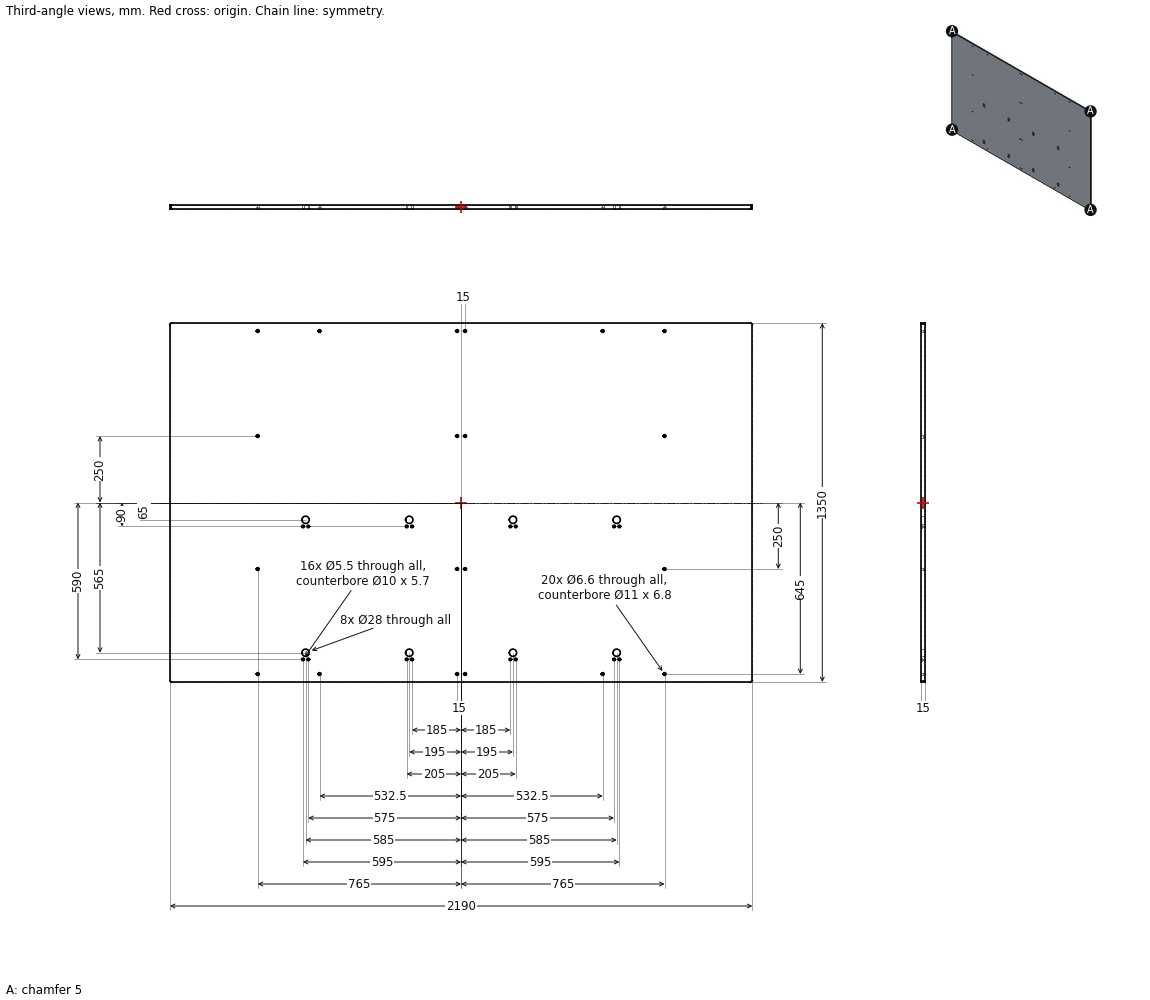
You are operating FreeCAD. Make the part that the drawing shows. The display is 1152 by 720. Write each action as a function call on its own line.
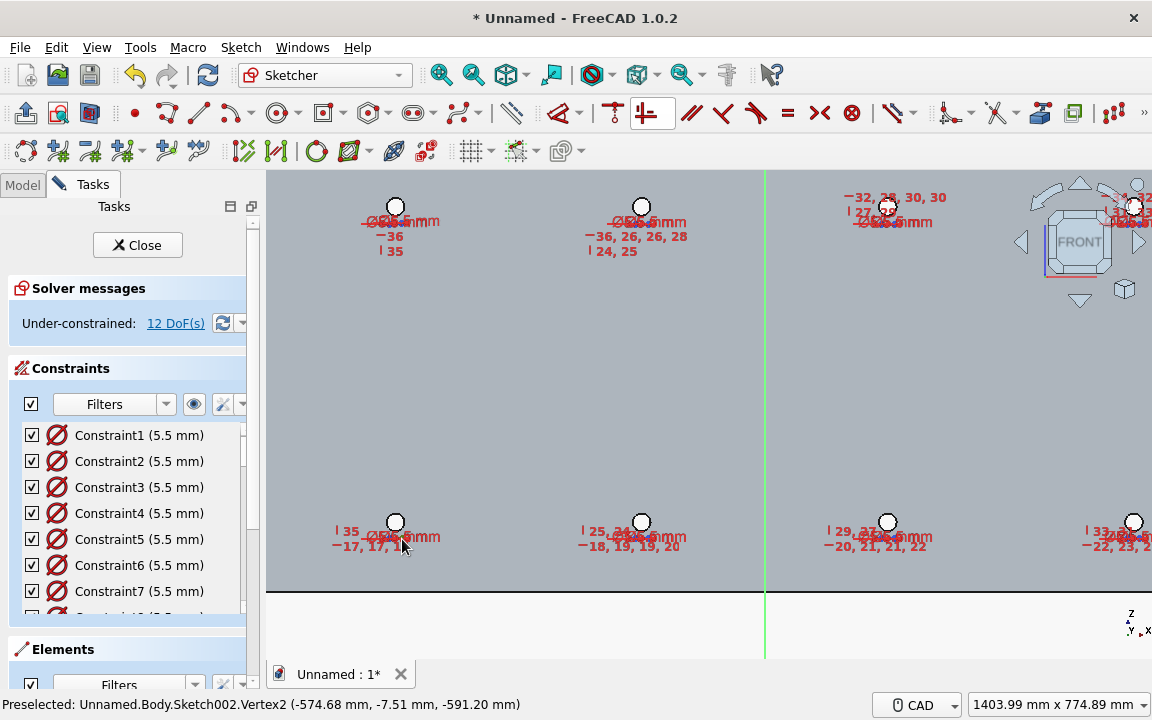
click(402, 223)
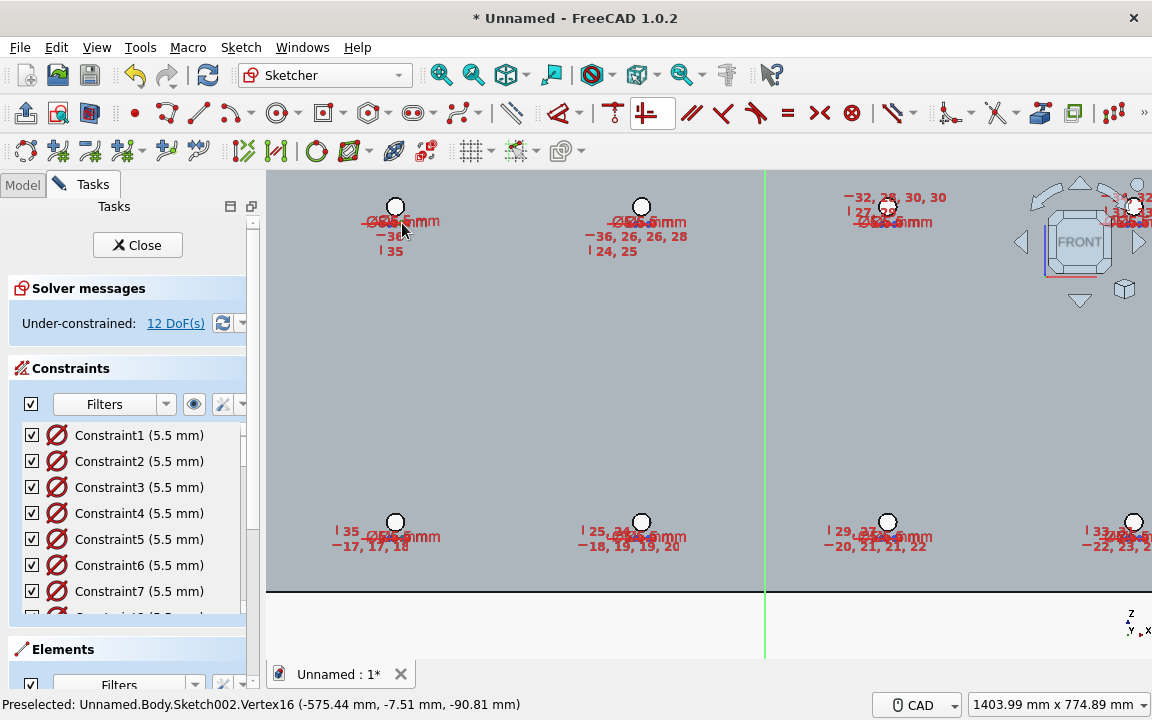
key(v)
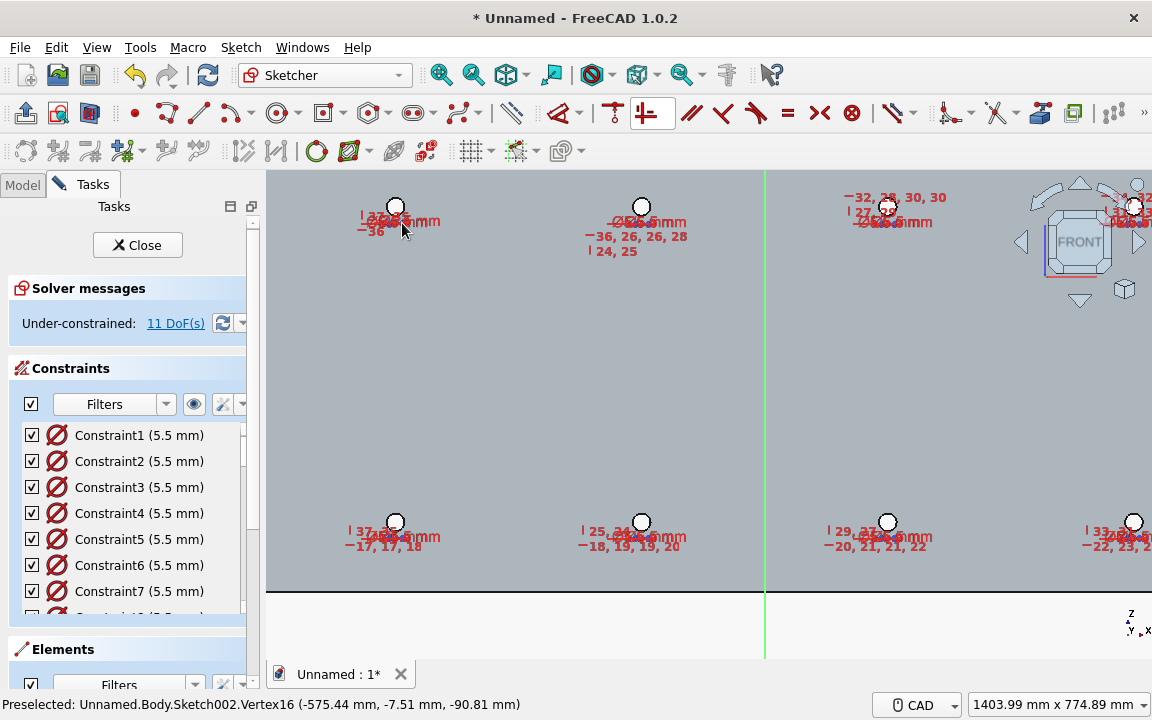
scroll(389, 224, up, 4)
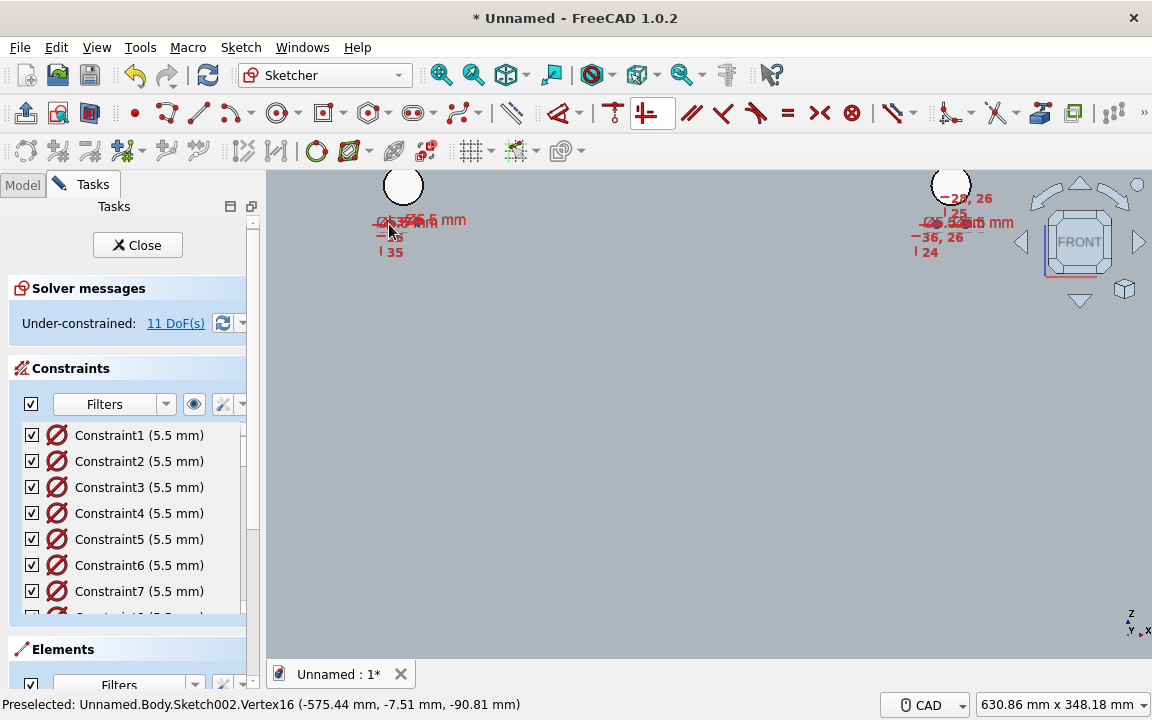
scroll(390, 225, up, 4)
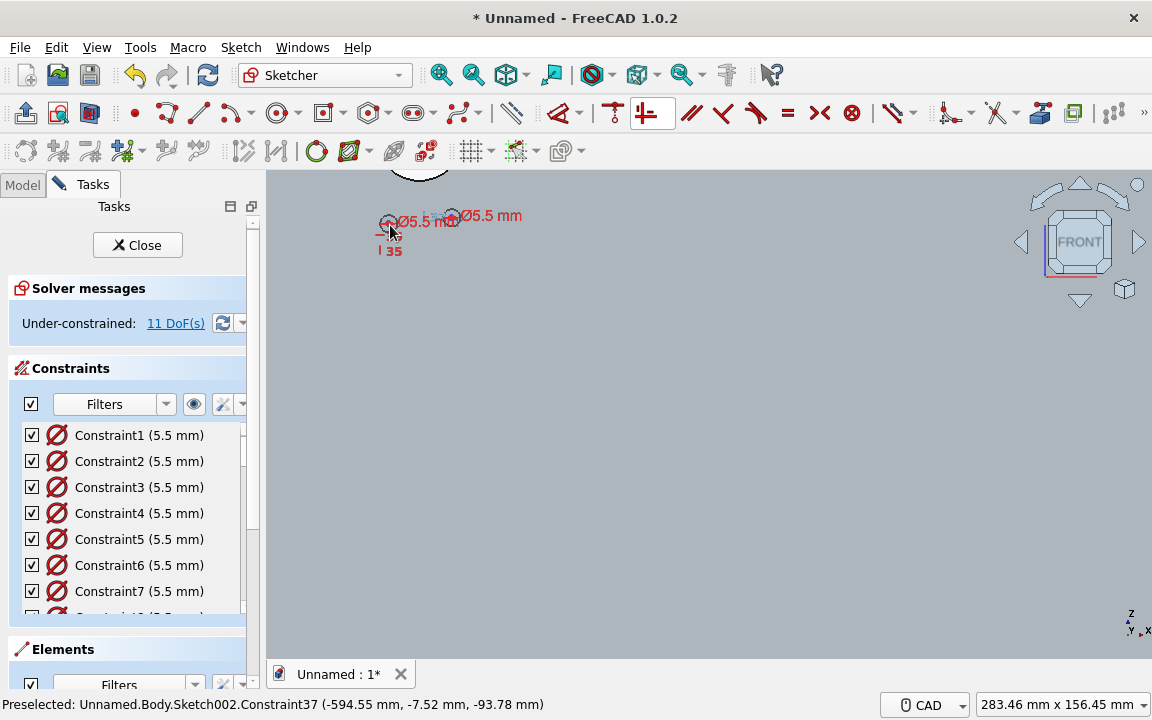
click(389, 224)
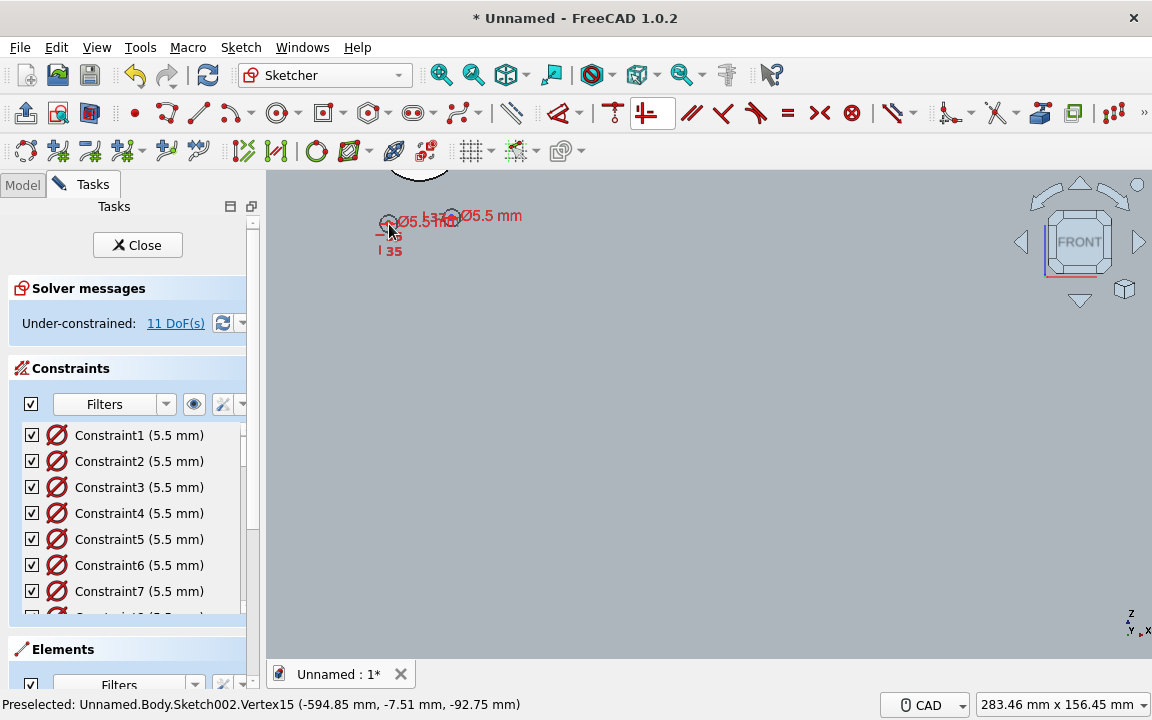
scroll(389, 345, down, 10)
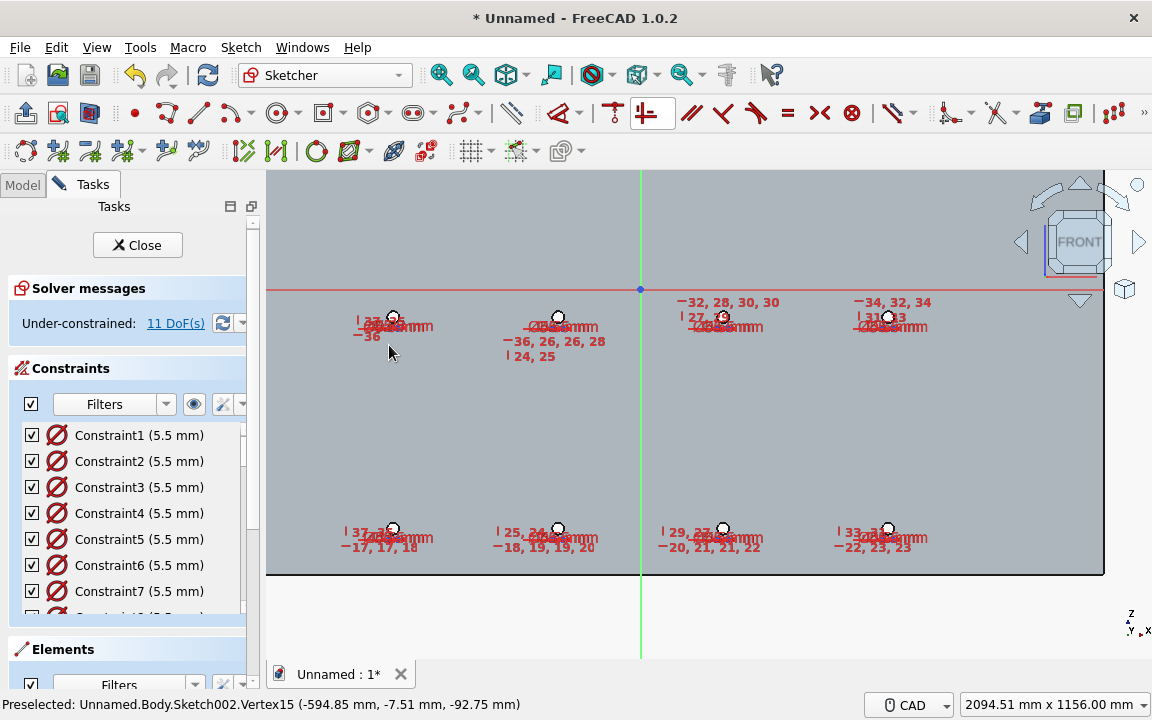
scroll(398, 328, up, 2)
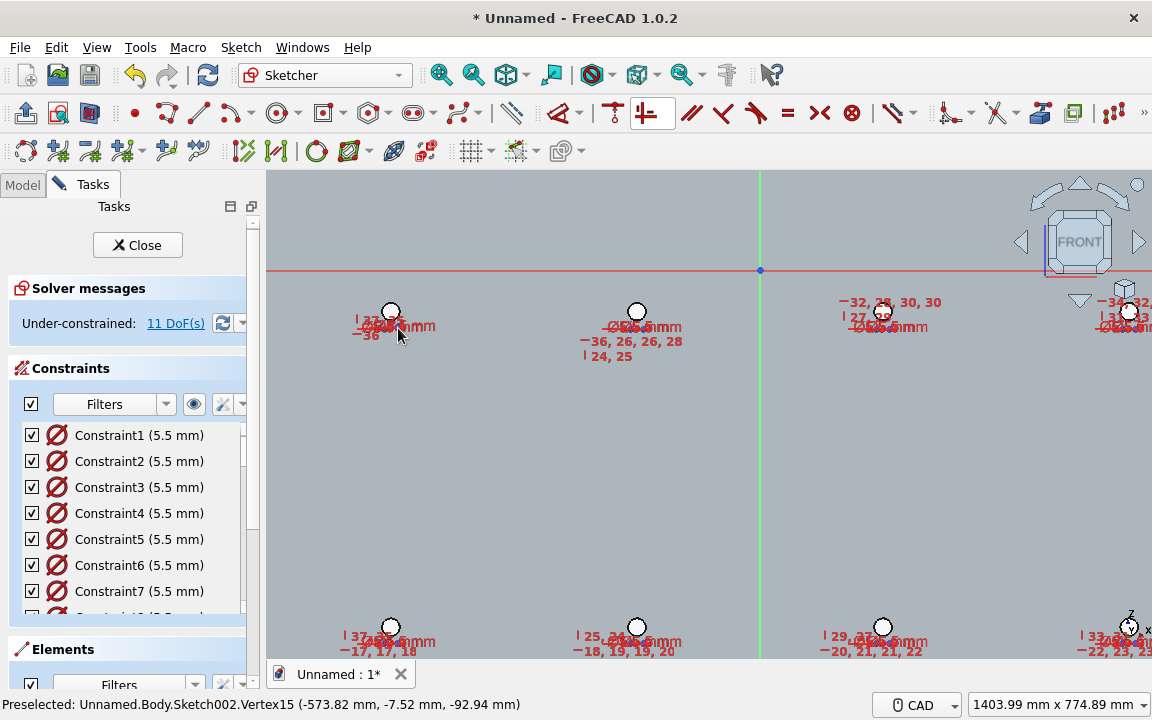
scroll(397, 328, up, 4)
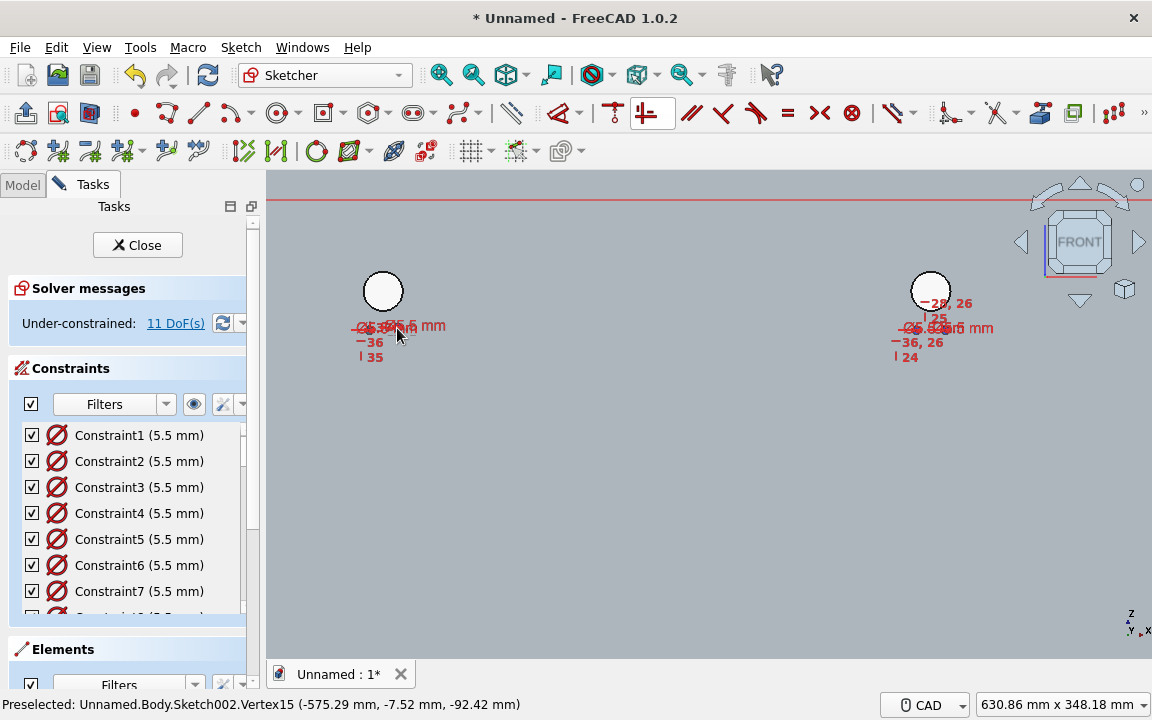
click(398, 328)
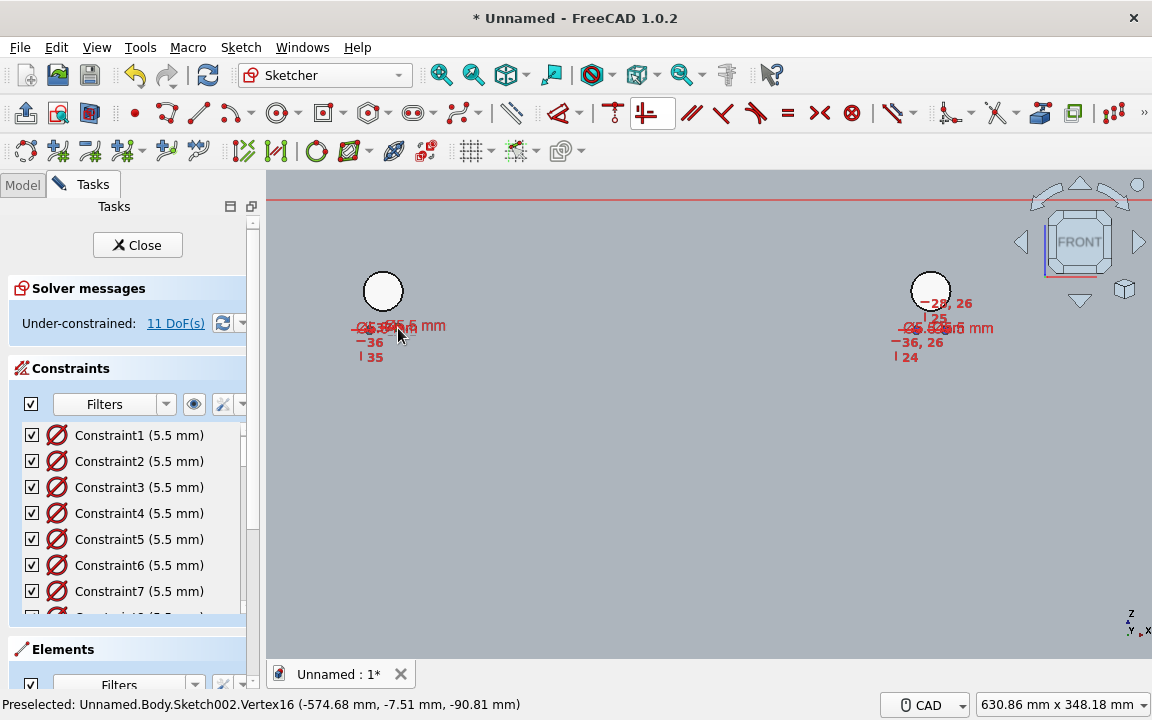
click(670, 114)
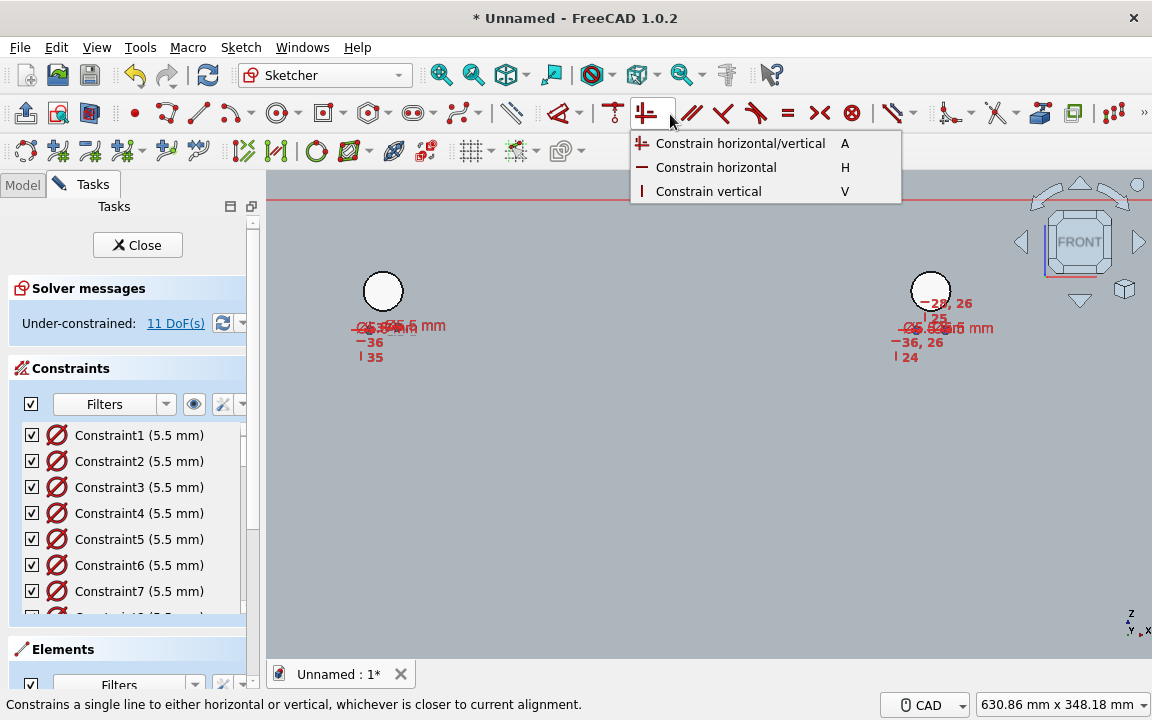
click(766, 167)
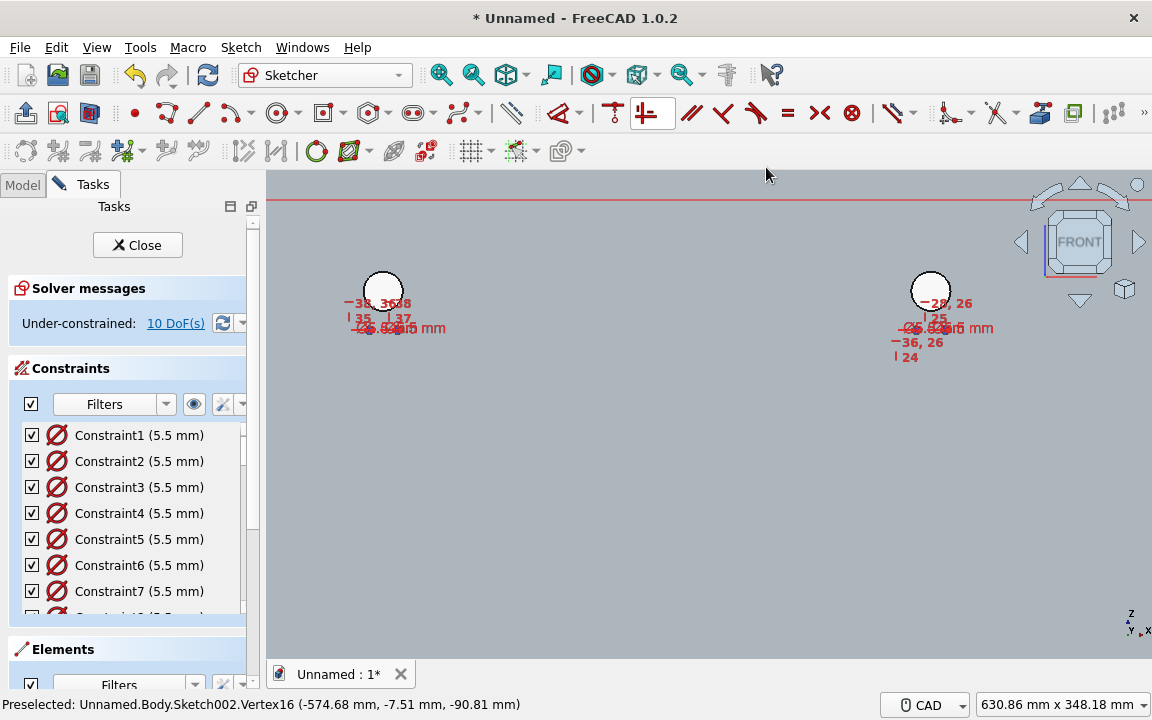
key(d)